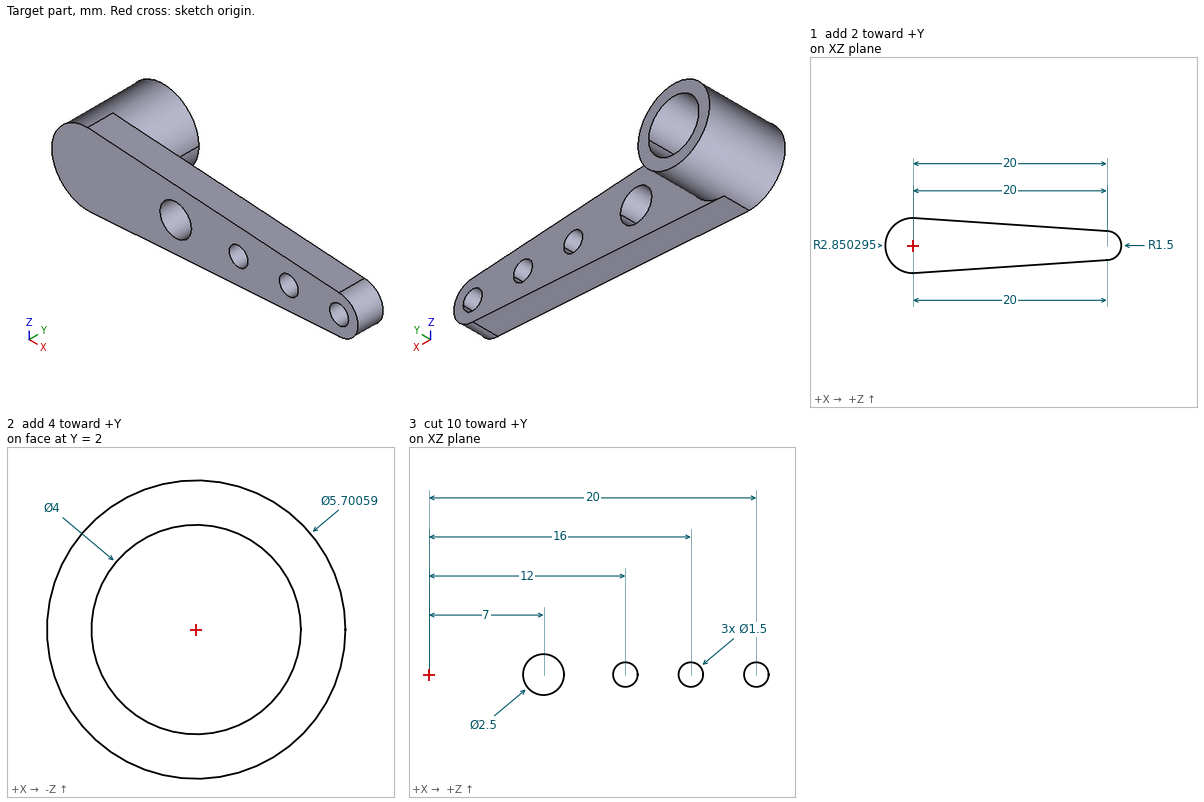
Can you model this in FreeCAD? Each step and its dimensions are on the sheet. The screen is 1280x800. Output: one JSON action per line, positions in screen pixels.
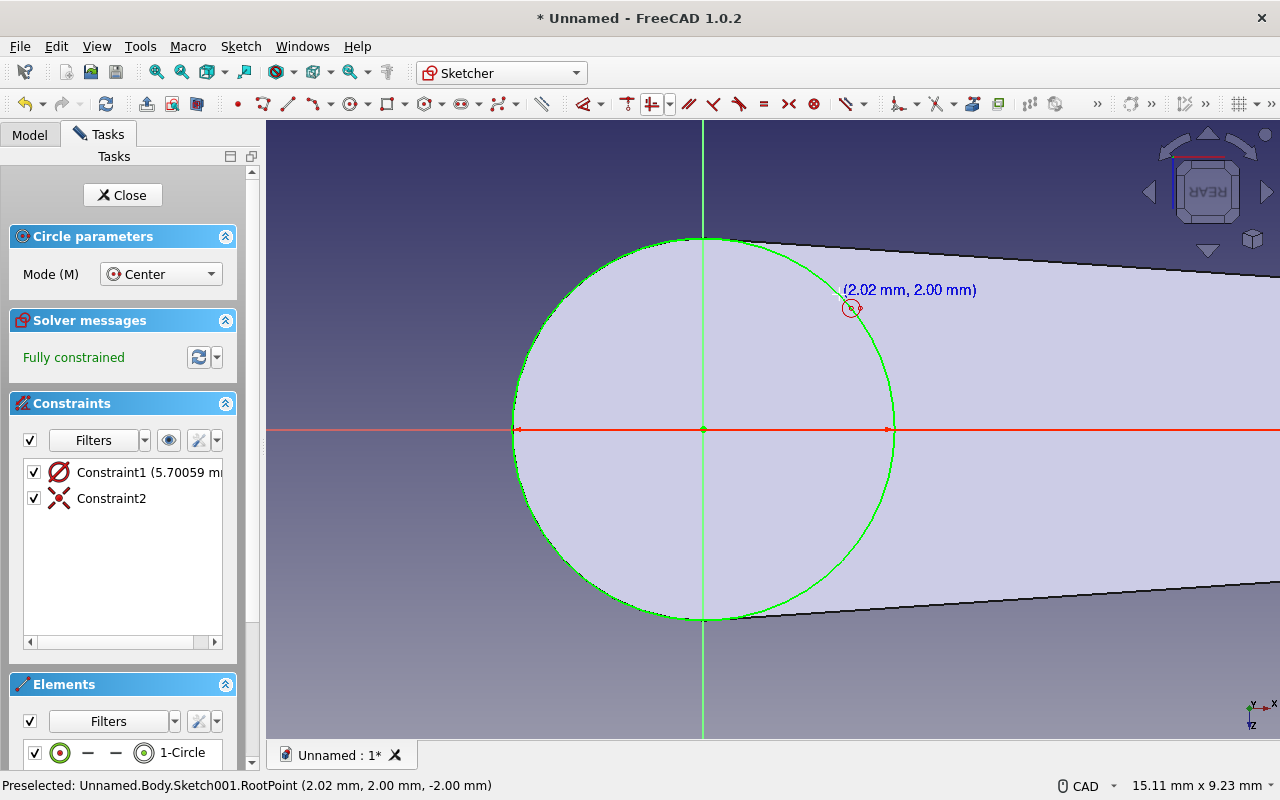
{"action": "left_click", "coordinate": [703, 429]}
{"action": "mouse_move", "coordinate": [798, 335]}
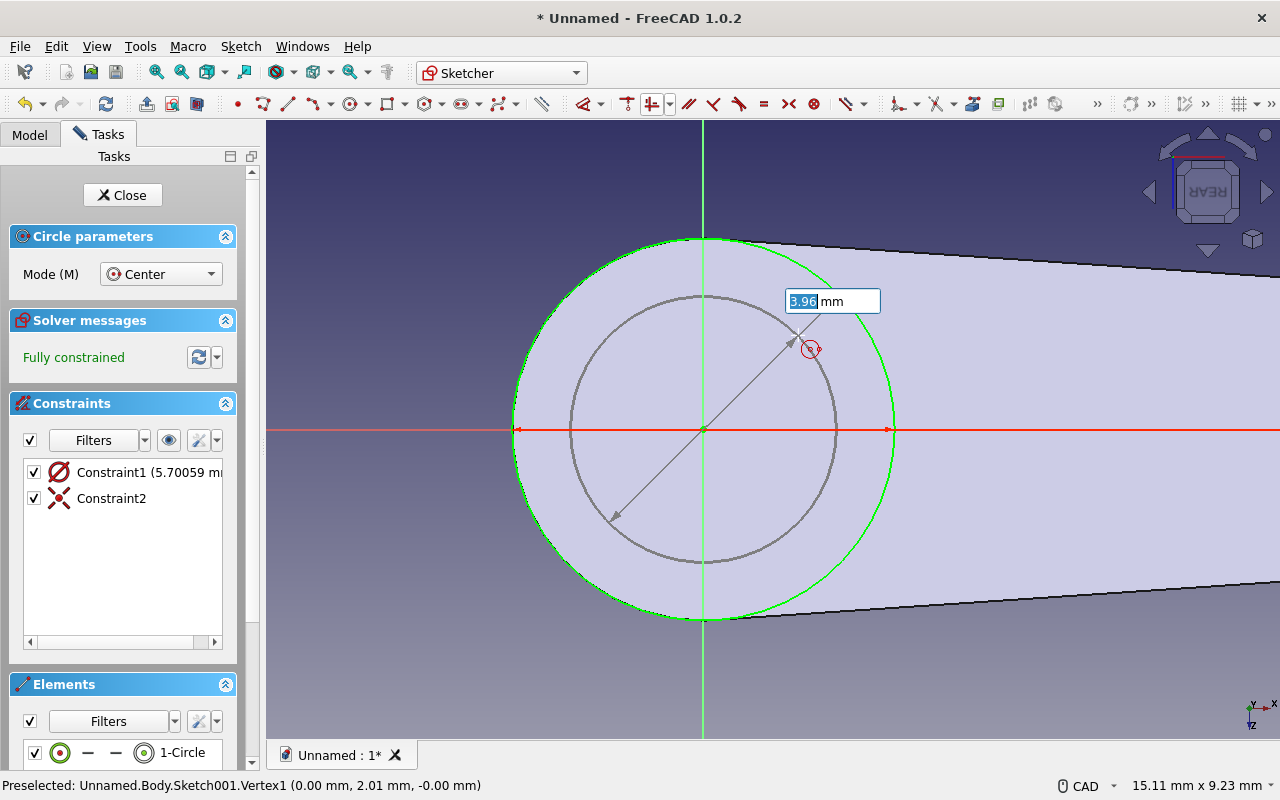
{"action": "type", "text": "4"}
{"action": "key", "text": "Return"}
{"action": "key", "text": "Escape"}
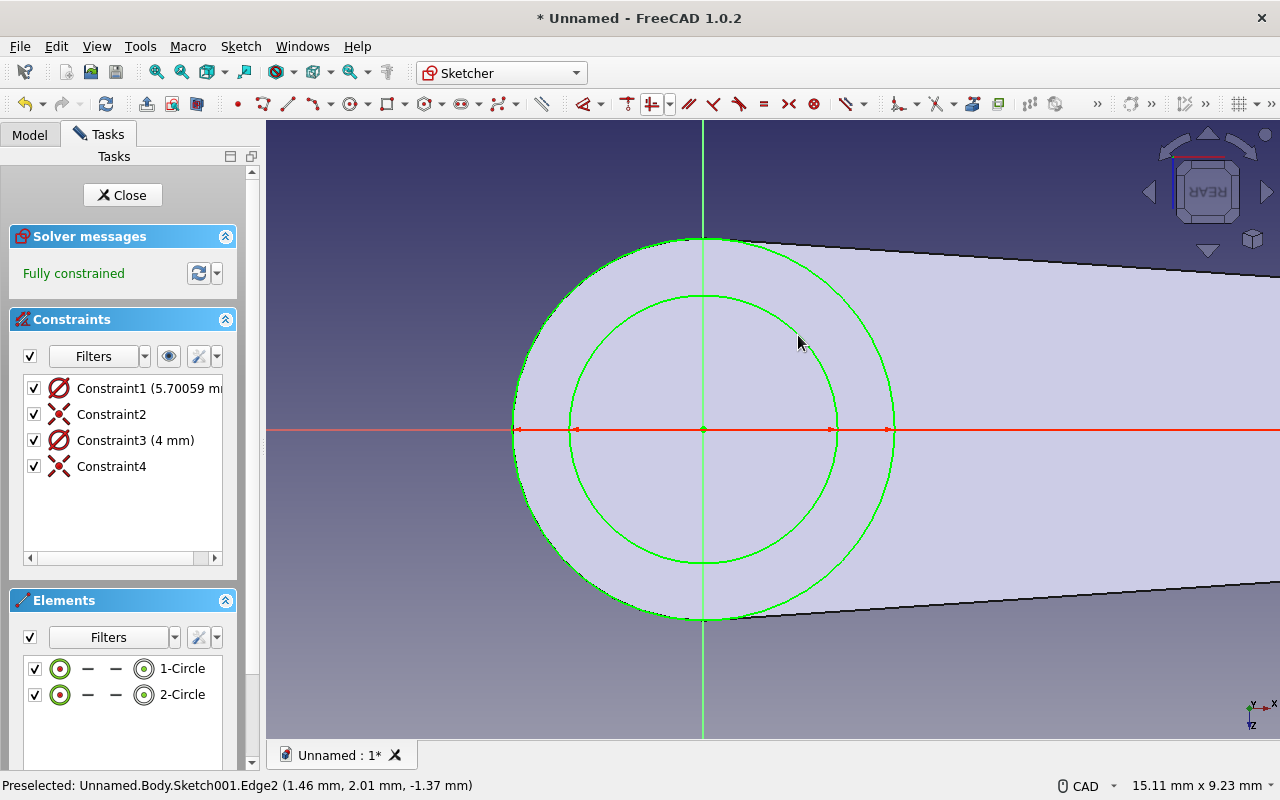
{"action": "left_click", "coordinate": [123, 195]}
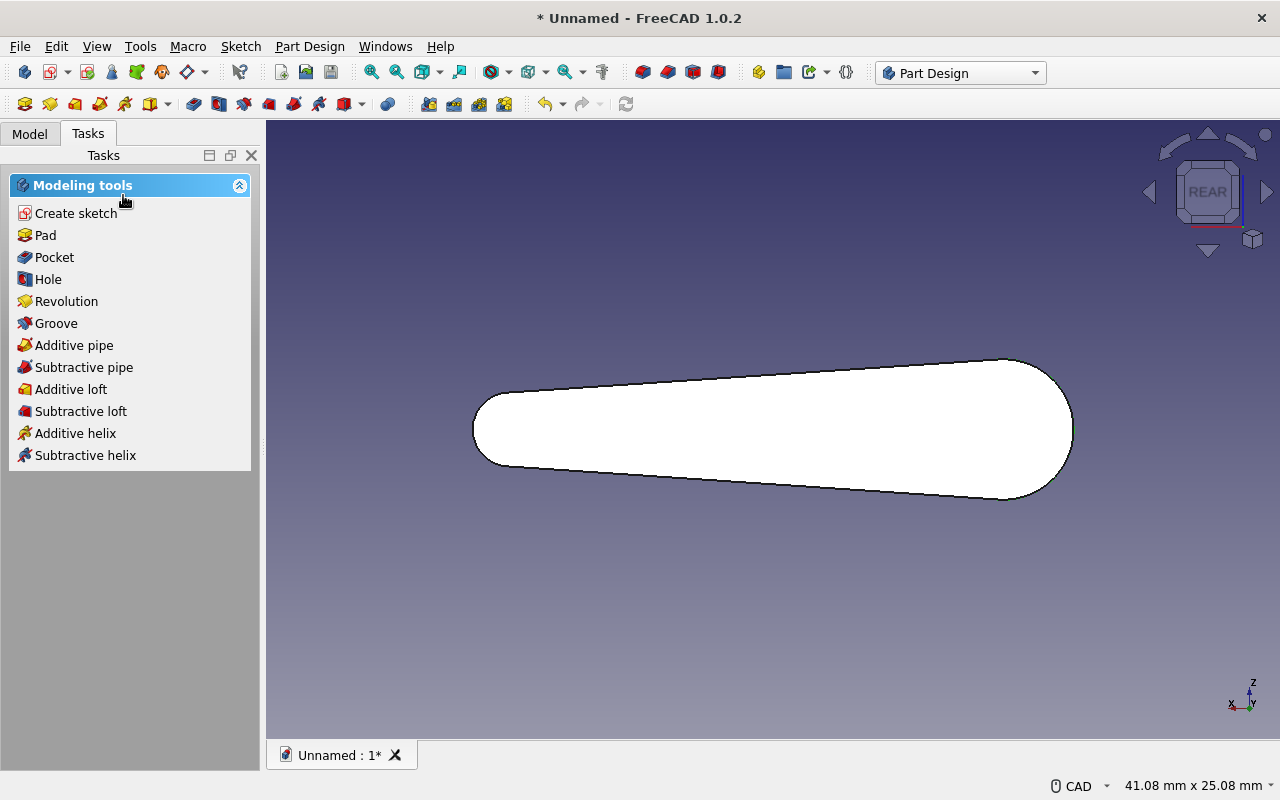
{"action": "left_click", "coordinate": [25, 104]}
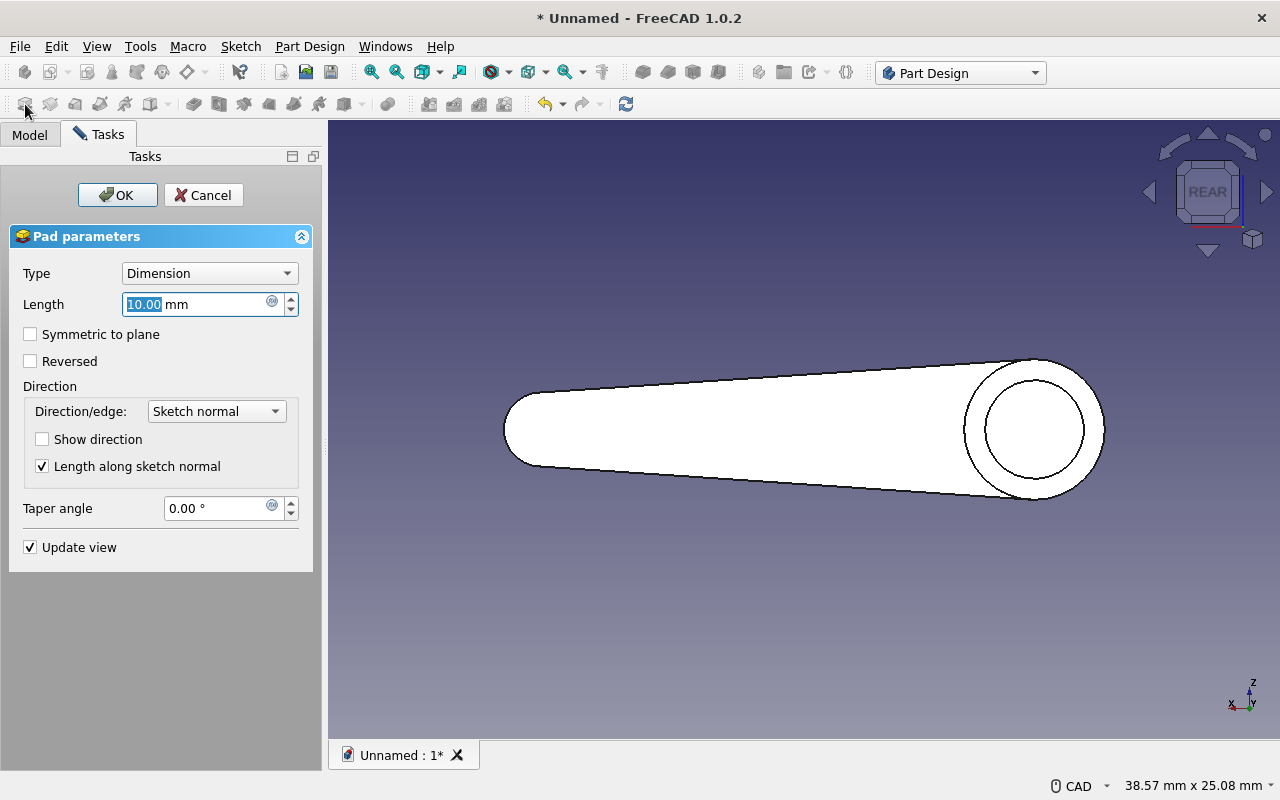
{"action": "type", "text": "4"}
{"action": "key", "text": "Tab"}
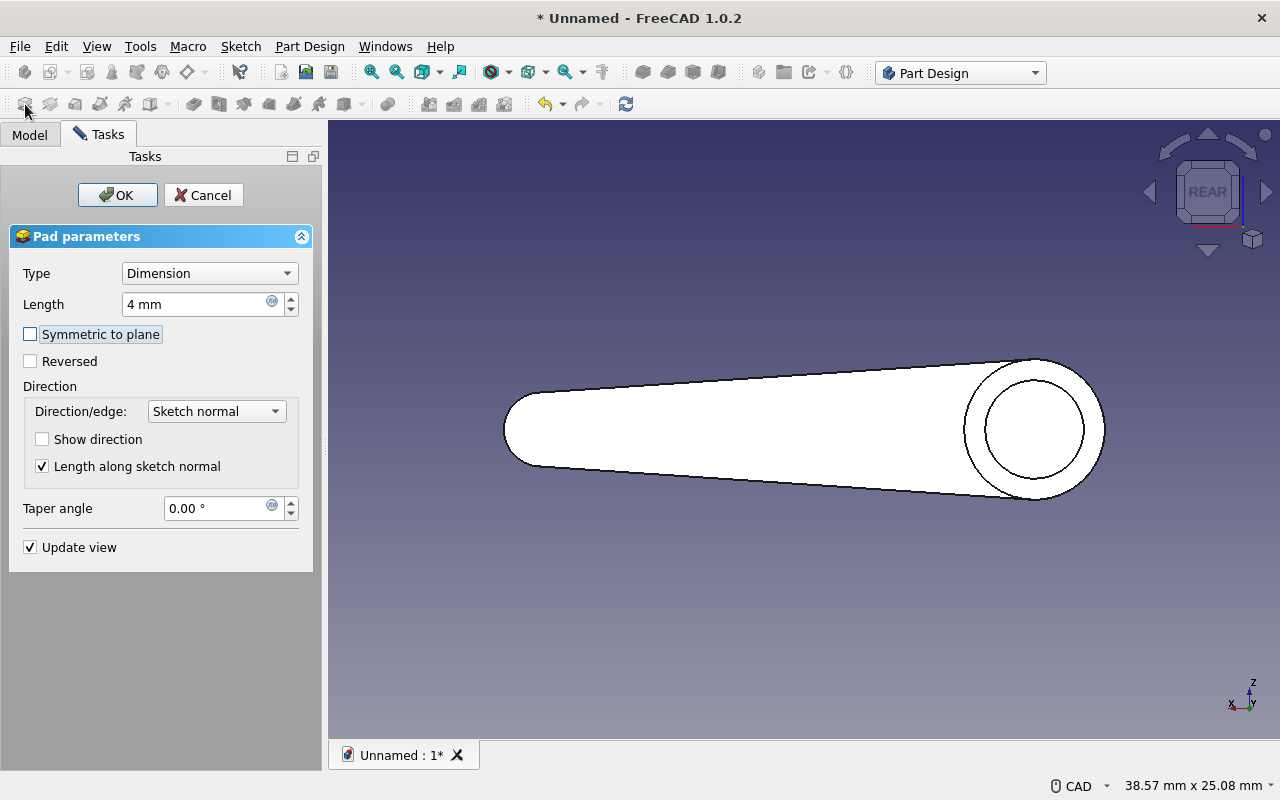
{"action": "left_click", "coordinate": [118, 195]}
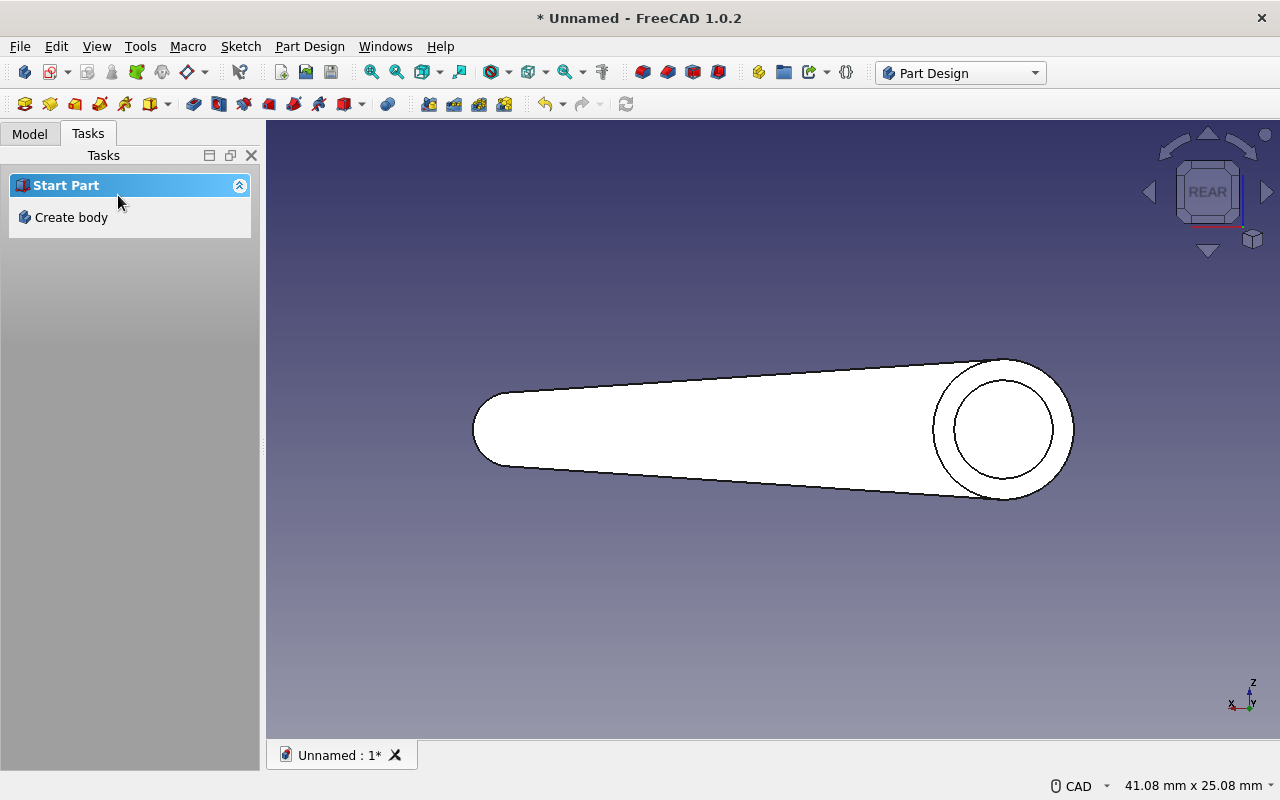
{"action": "left_click", "coordinate": [50, 72]}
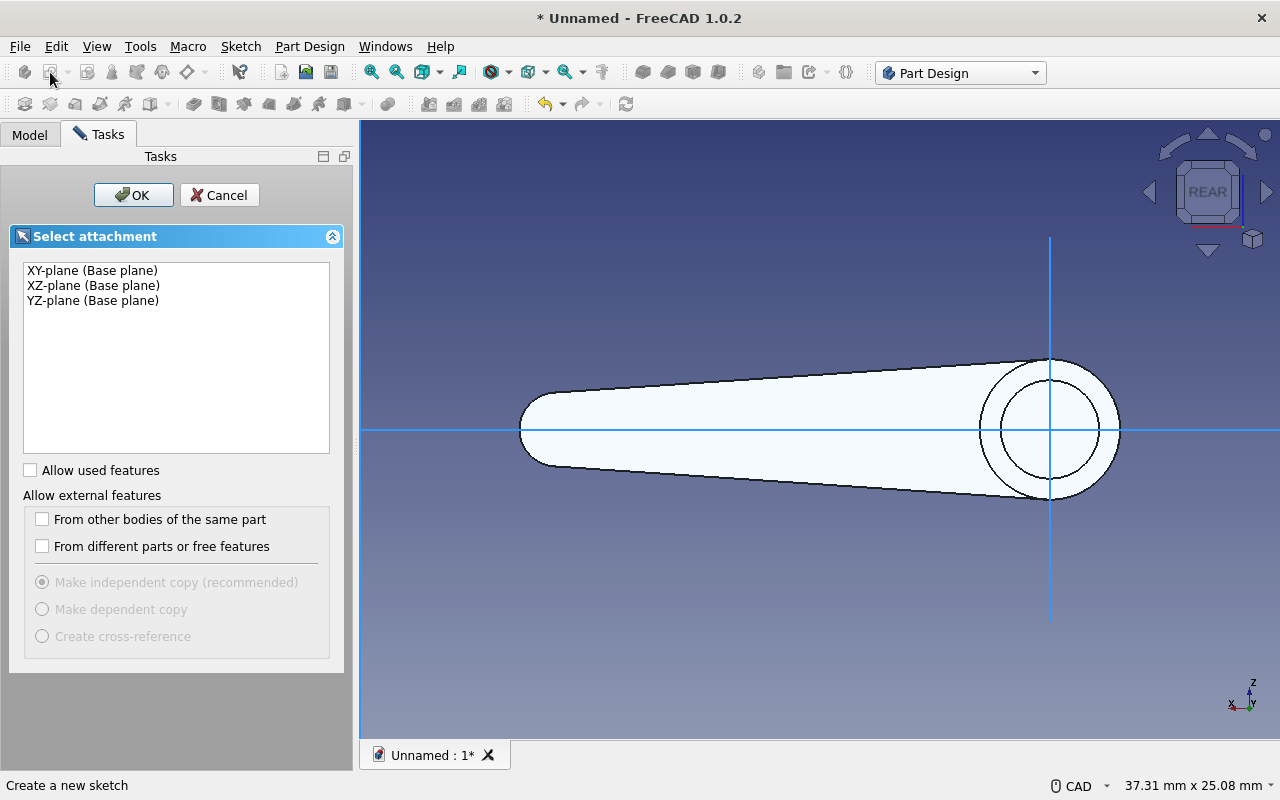
{"action": "left_click", "coordinate": [84, 286]}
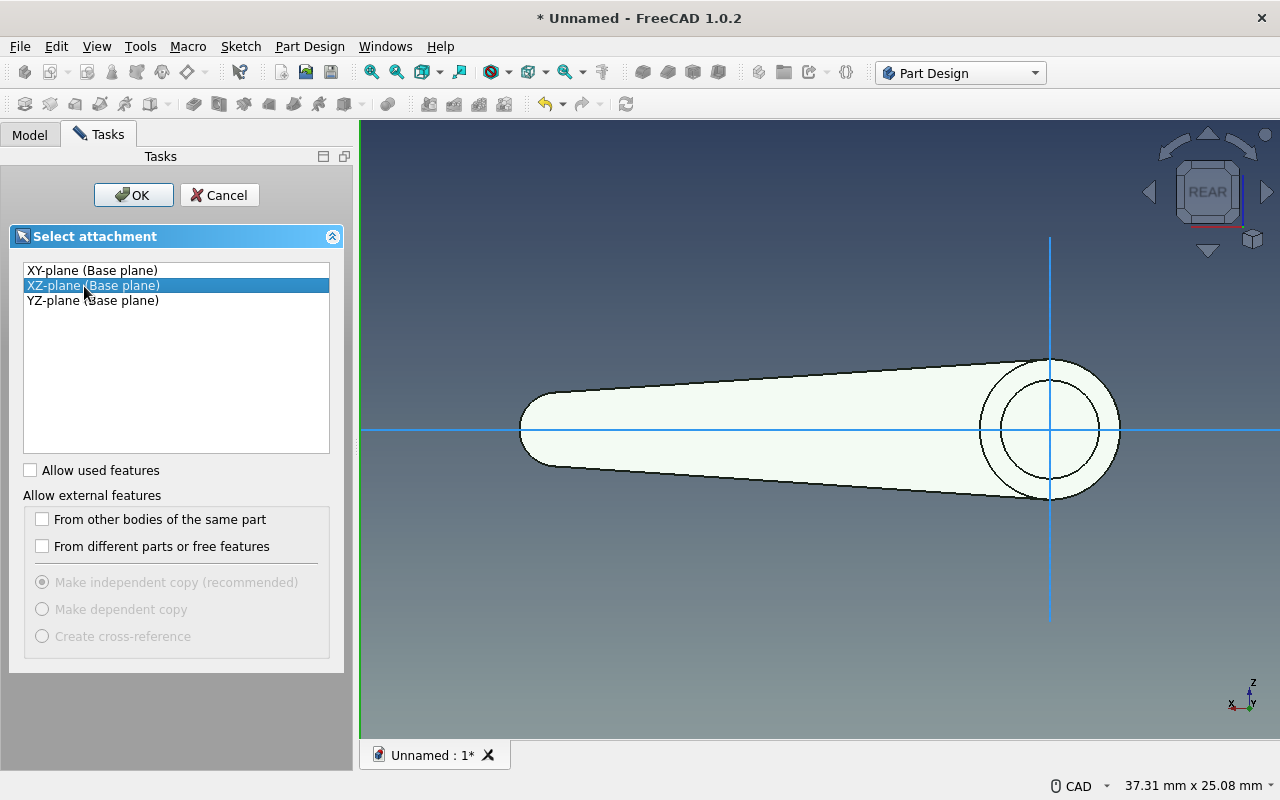
{"action": "left_click", "coordinate": [134, 195]}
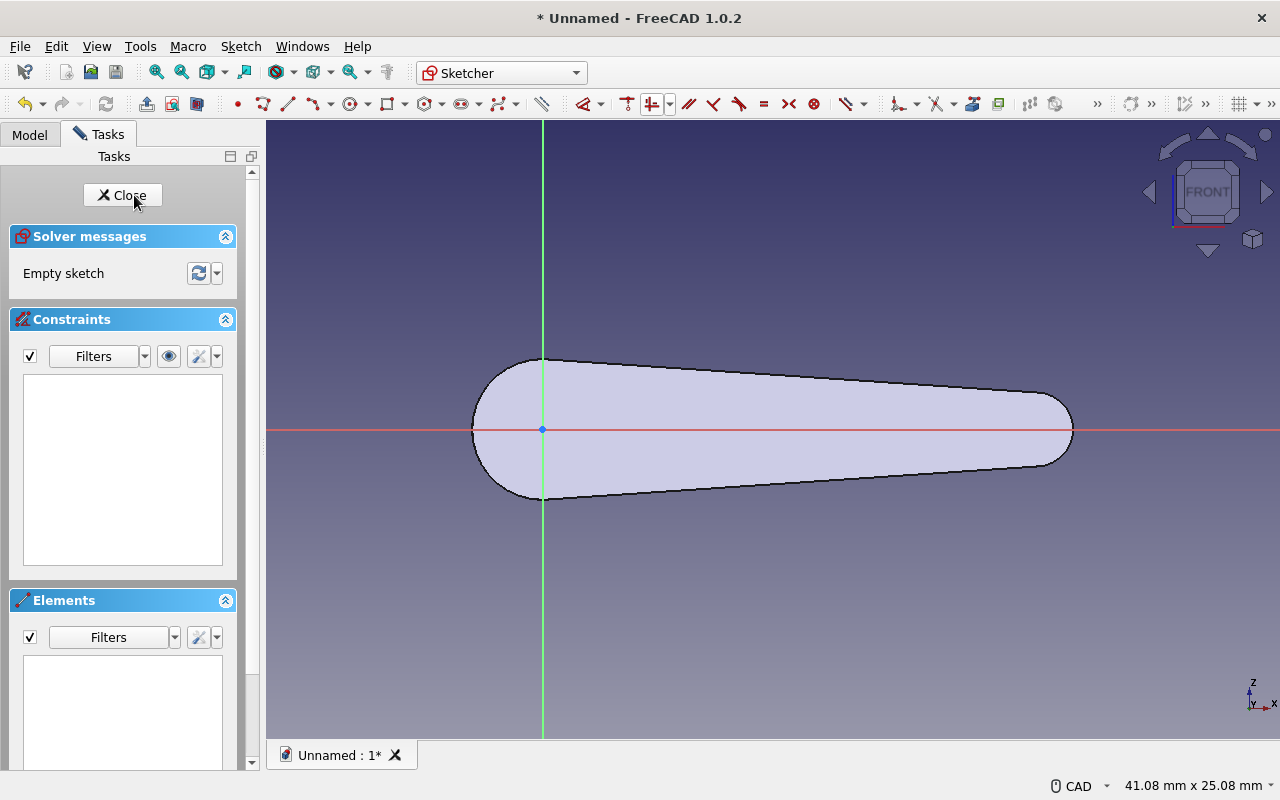
{"action": "left_click", "coordinate": [350, 104]}